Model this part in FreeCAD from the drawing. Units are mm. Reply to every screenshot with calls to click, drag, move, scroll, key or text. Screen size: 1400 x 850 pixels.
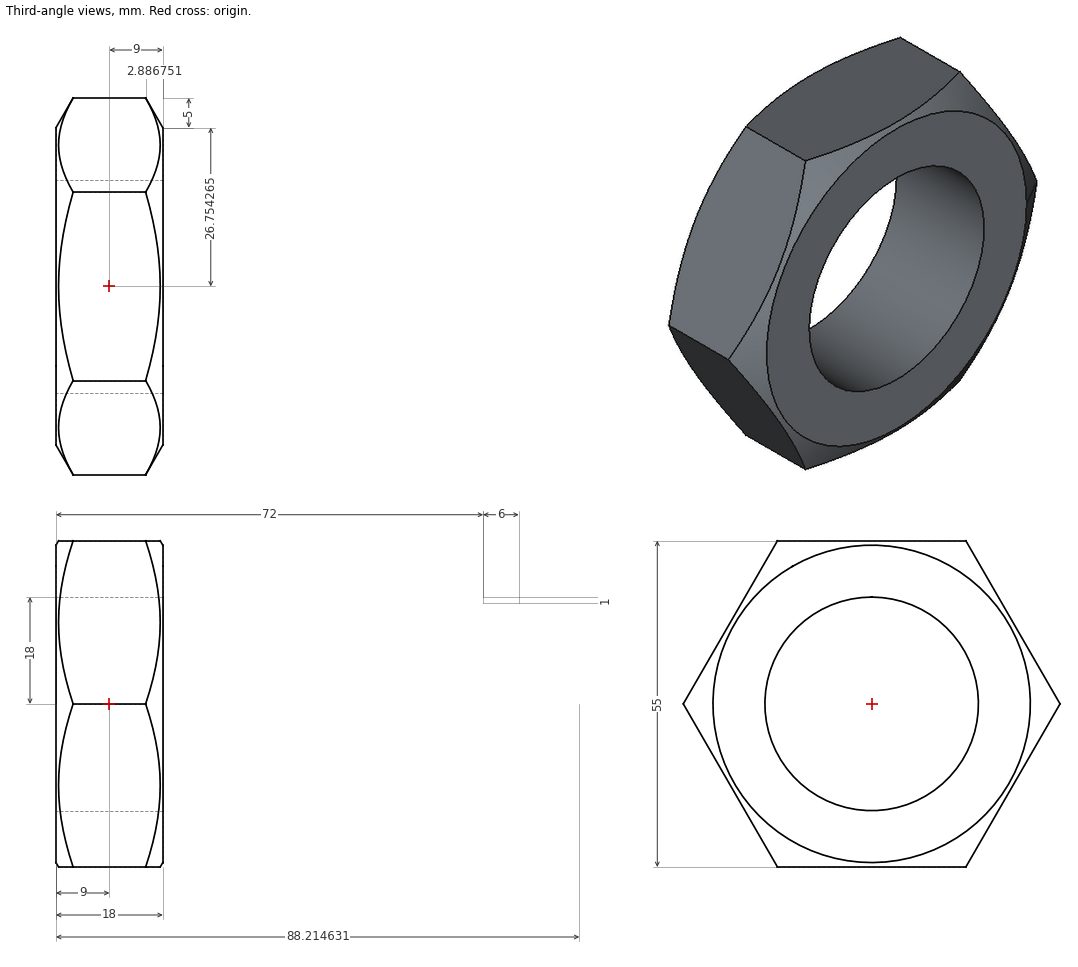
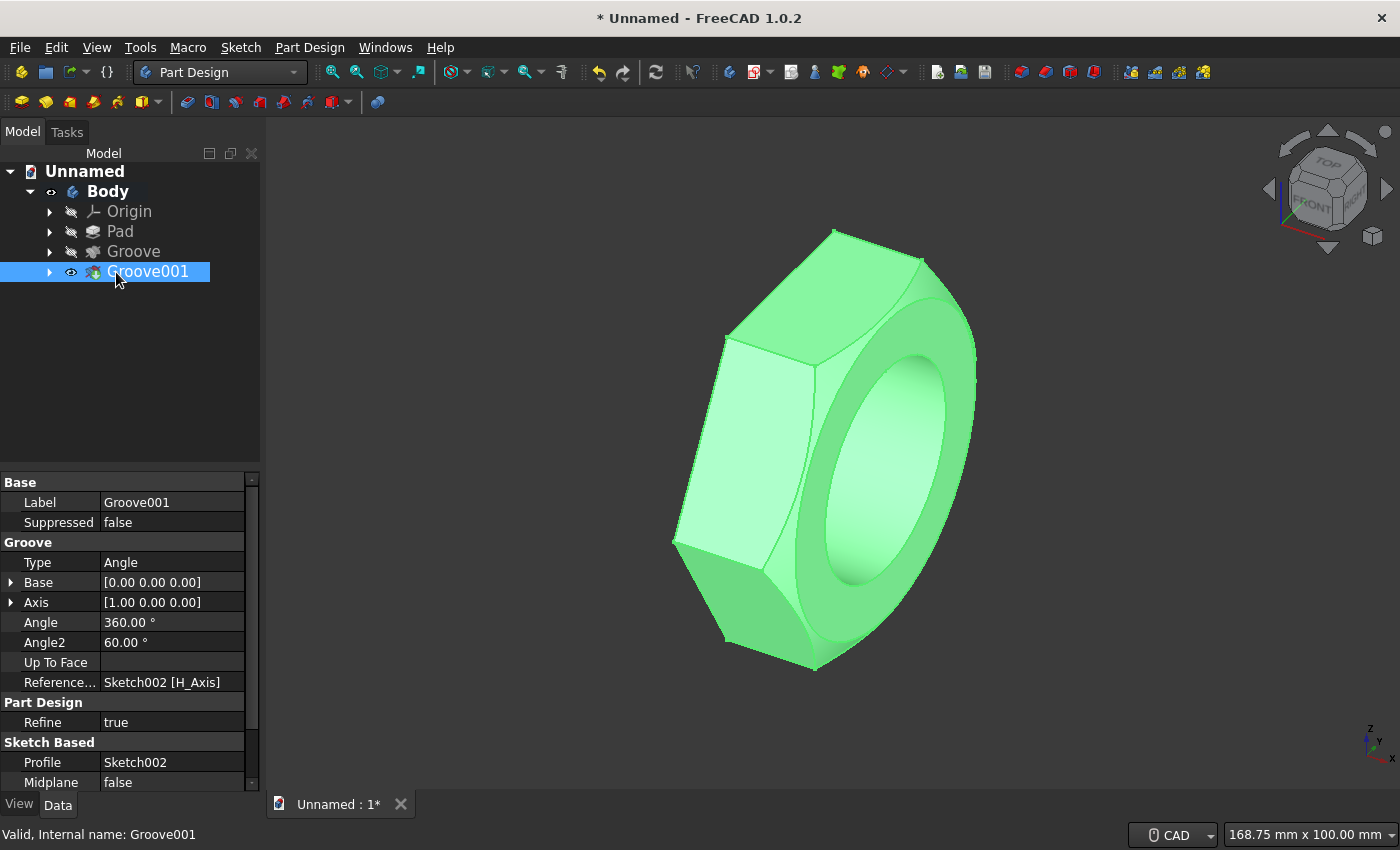
click(1132, 72)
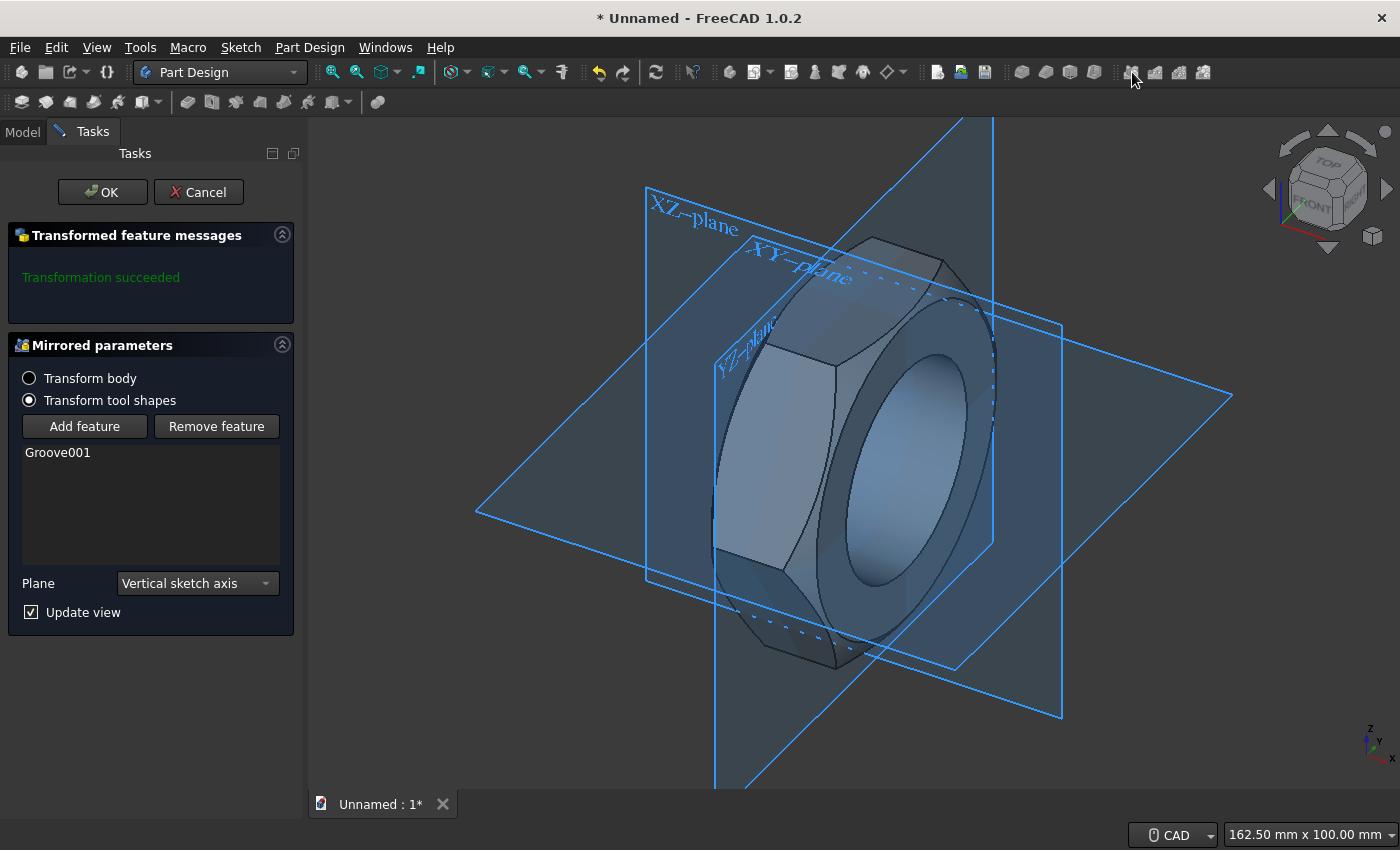
click(198, 584)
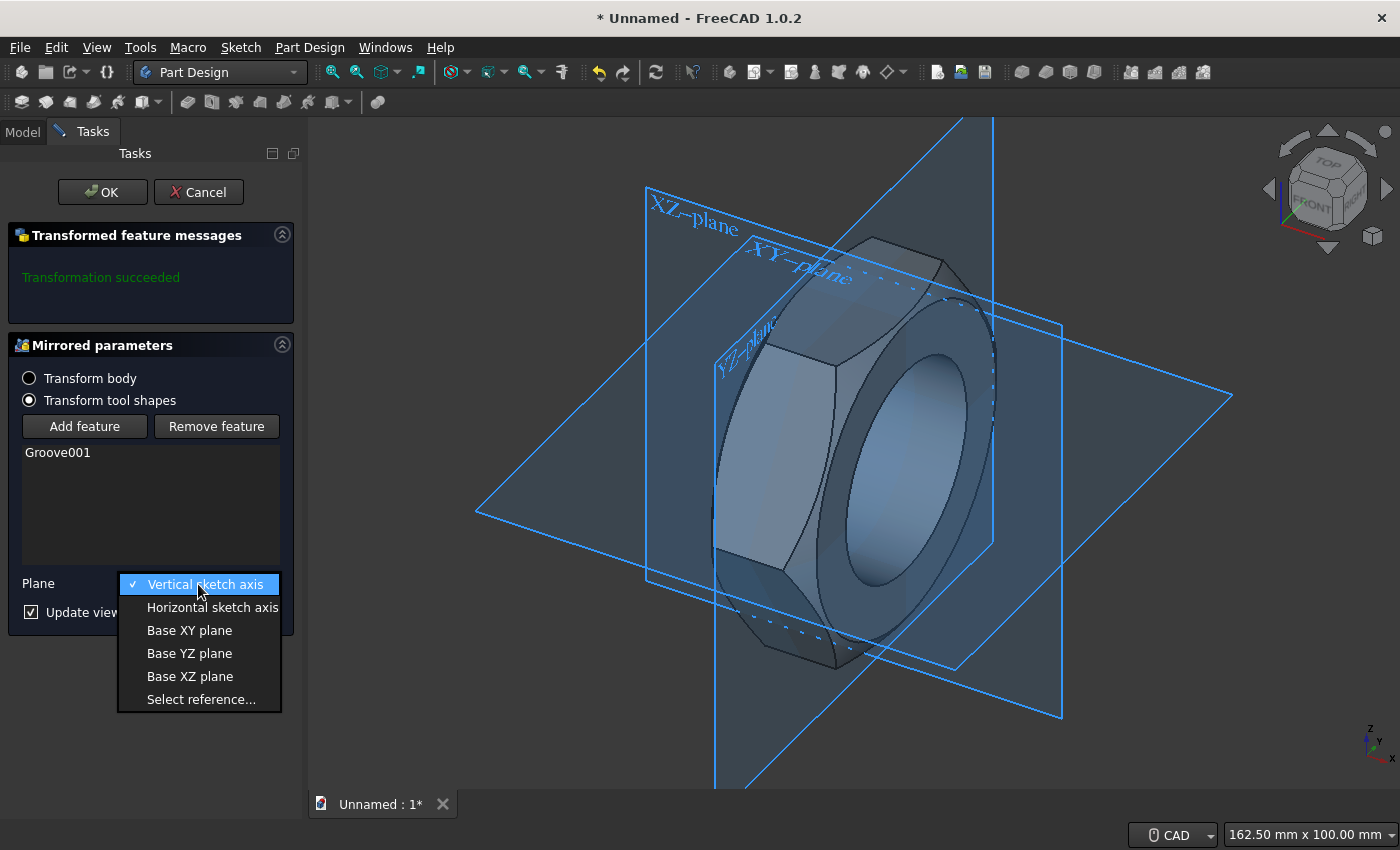
click(198, 654)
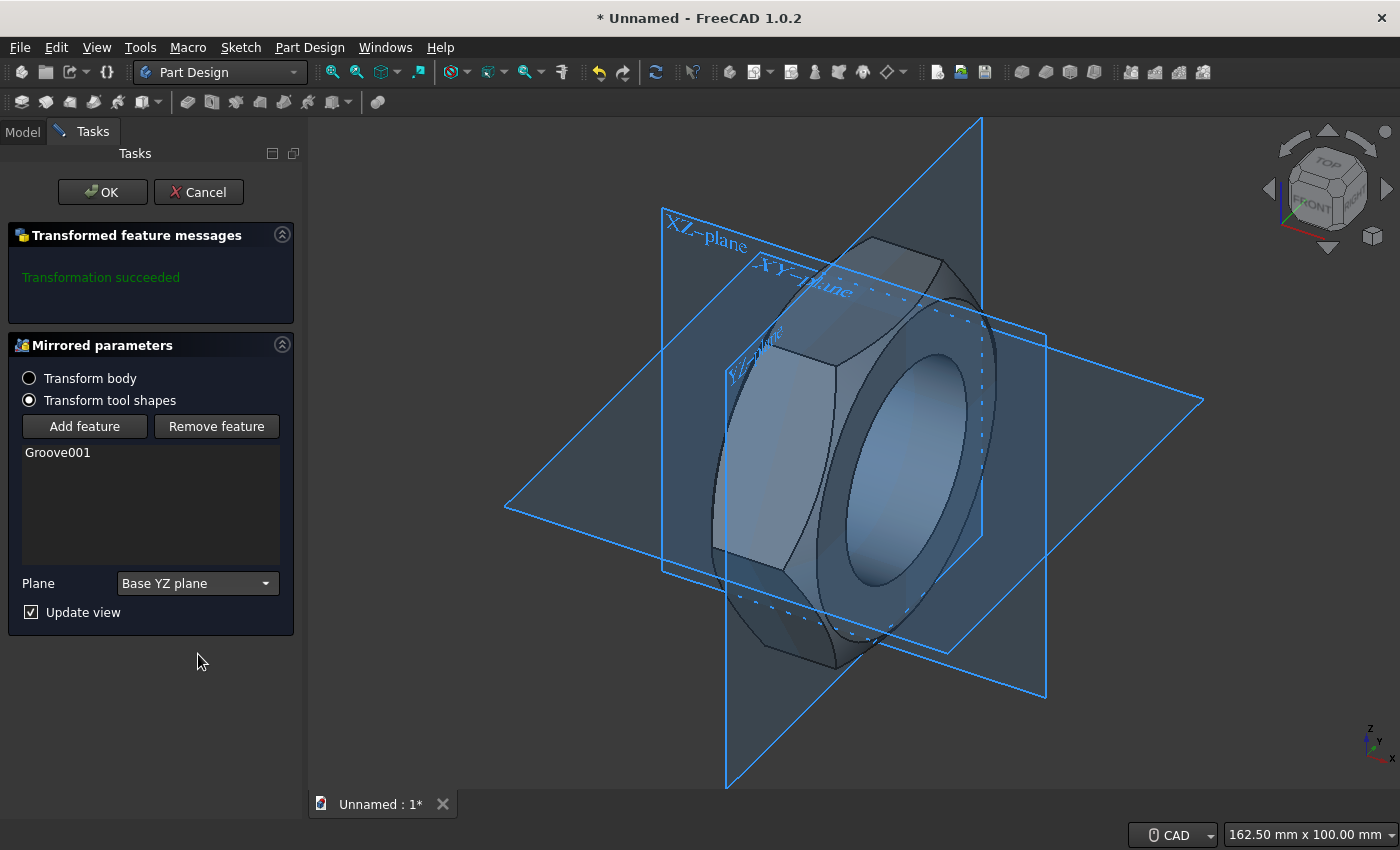
click(103, 192)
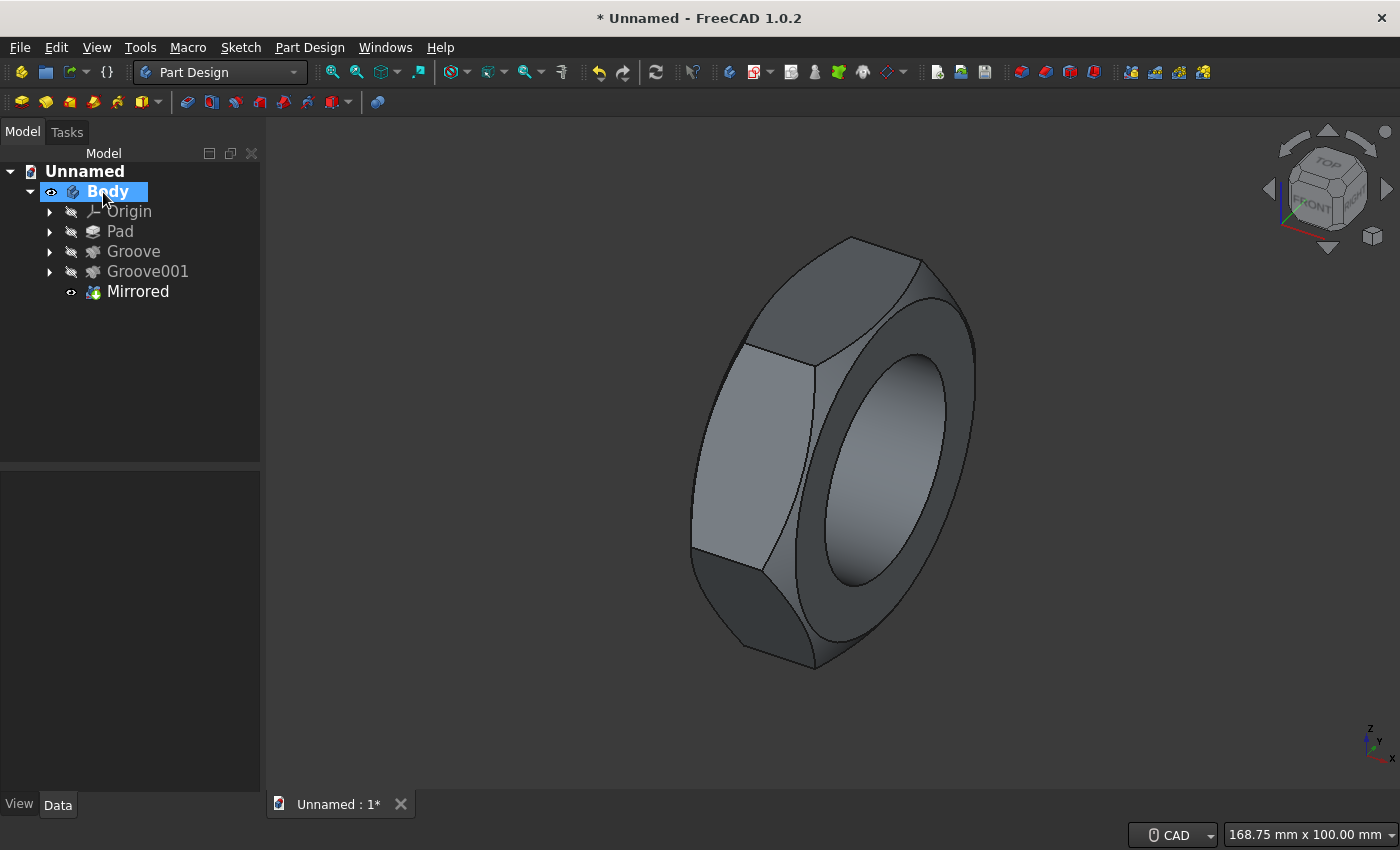
key(0)